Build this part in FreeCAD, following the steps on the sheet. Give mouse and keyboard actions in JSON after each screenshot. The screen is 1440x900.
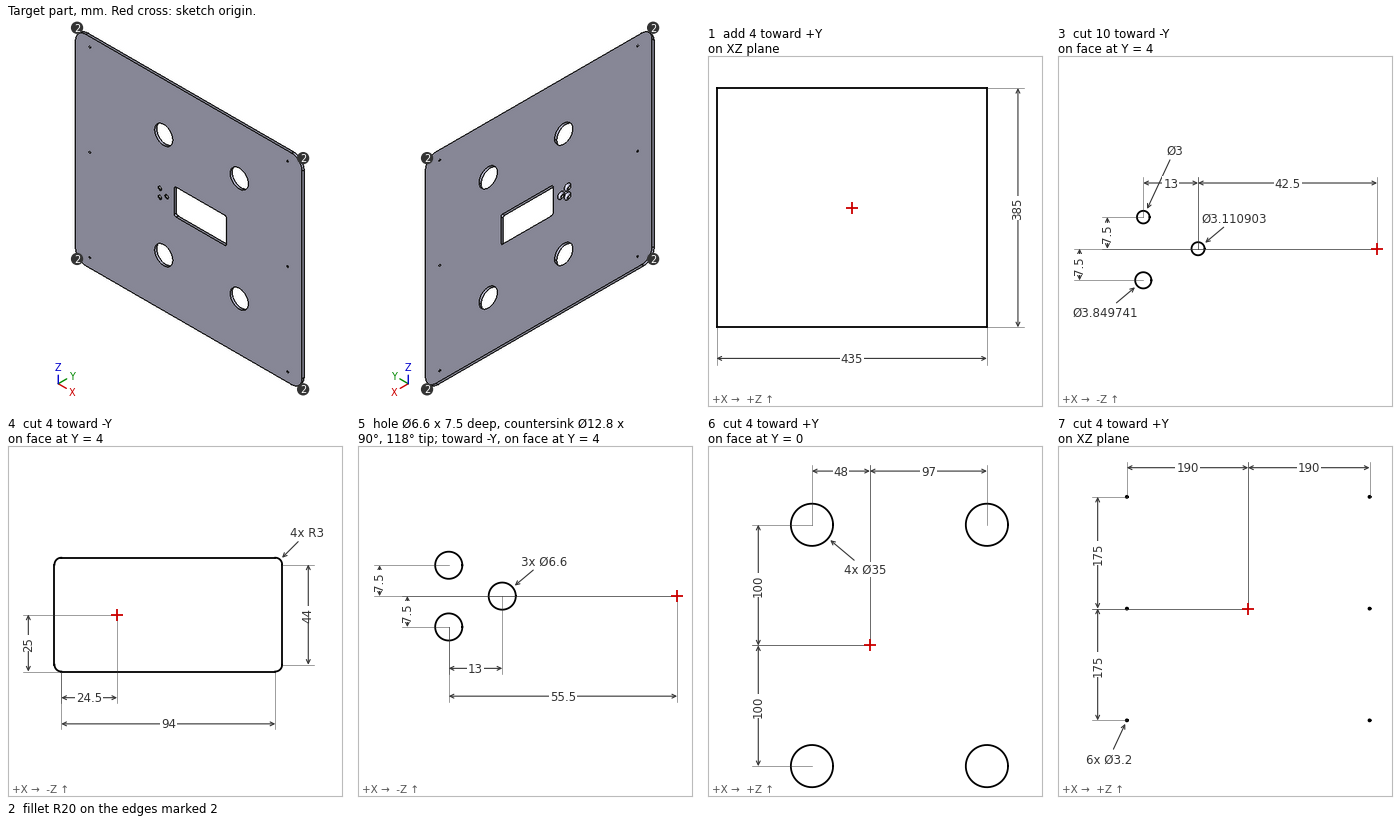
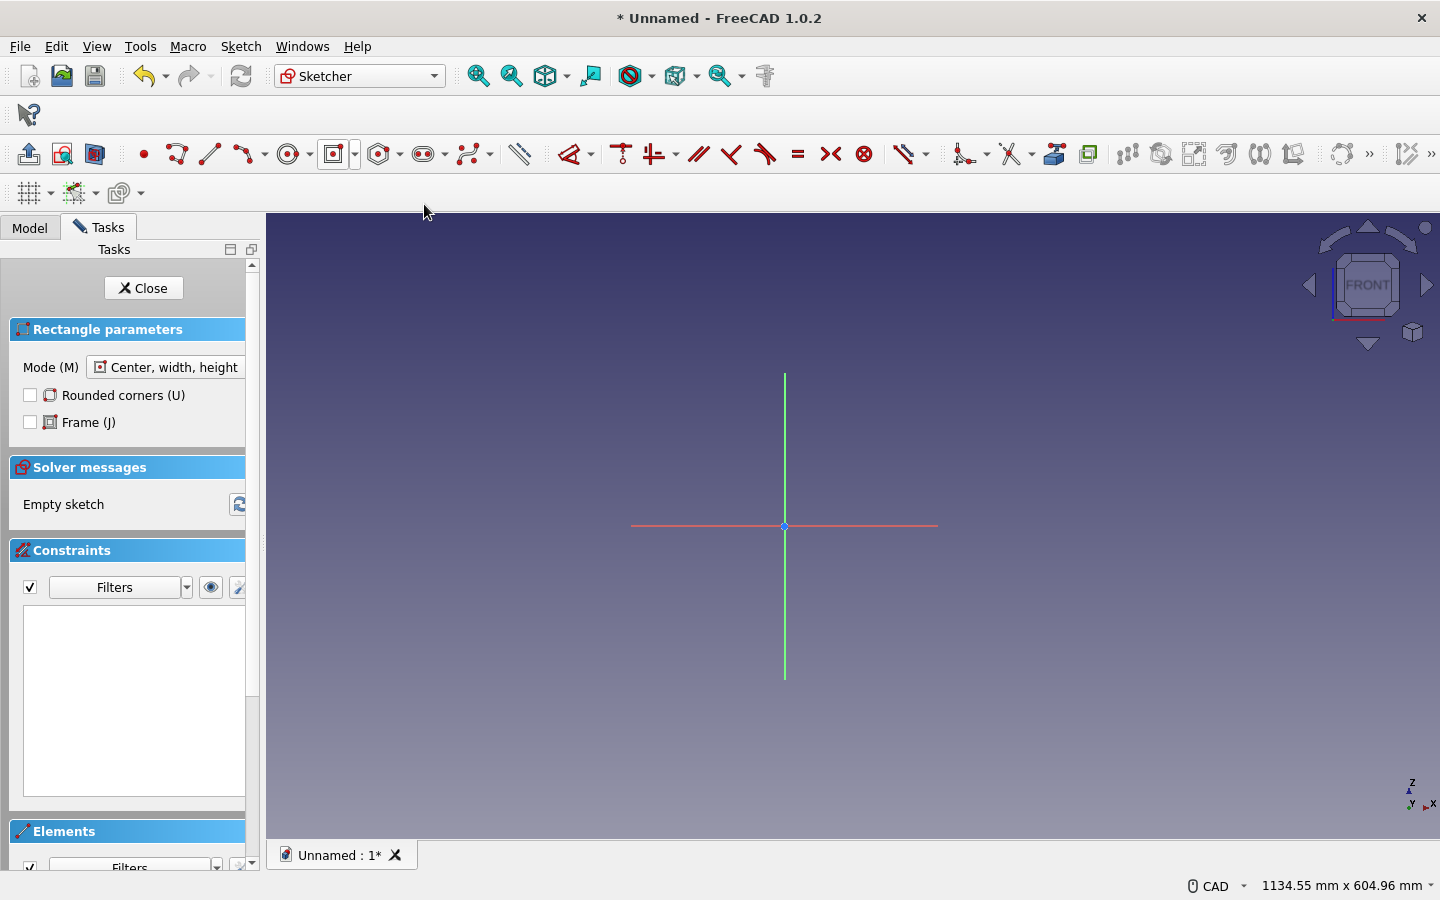
{"action": "left_click", "coordinate": [785, 526]}
{"action": "left_click", "coordinate": [1010, 327]}
{"action": "key", "text": "Escape"}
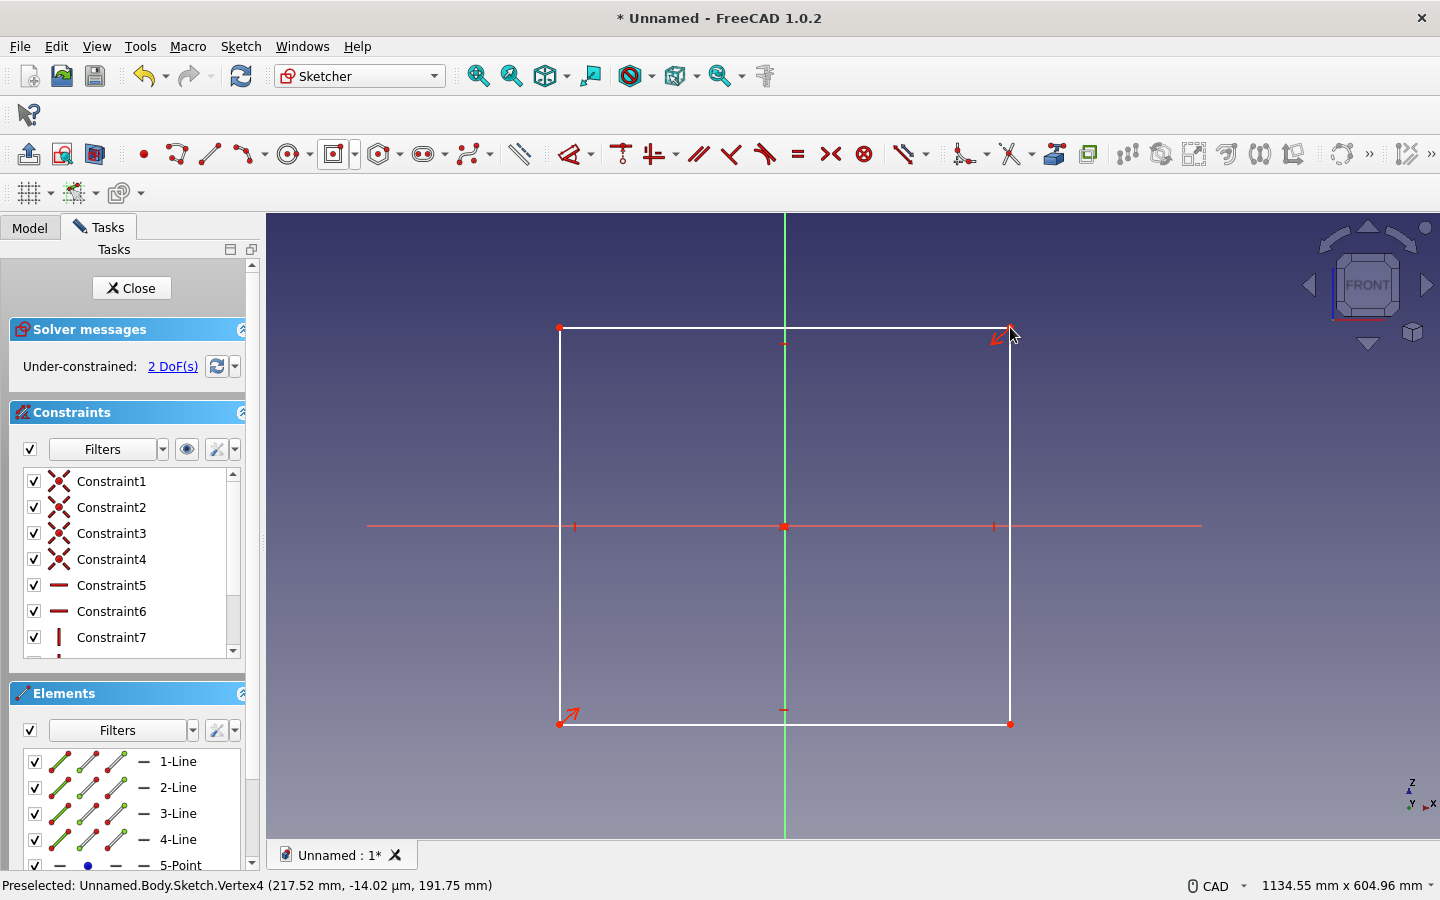
{"action": "left_click", "coordinate": [568, 154]}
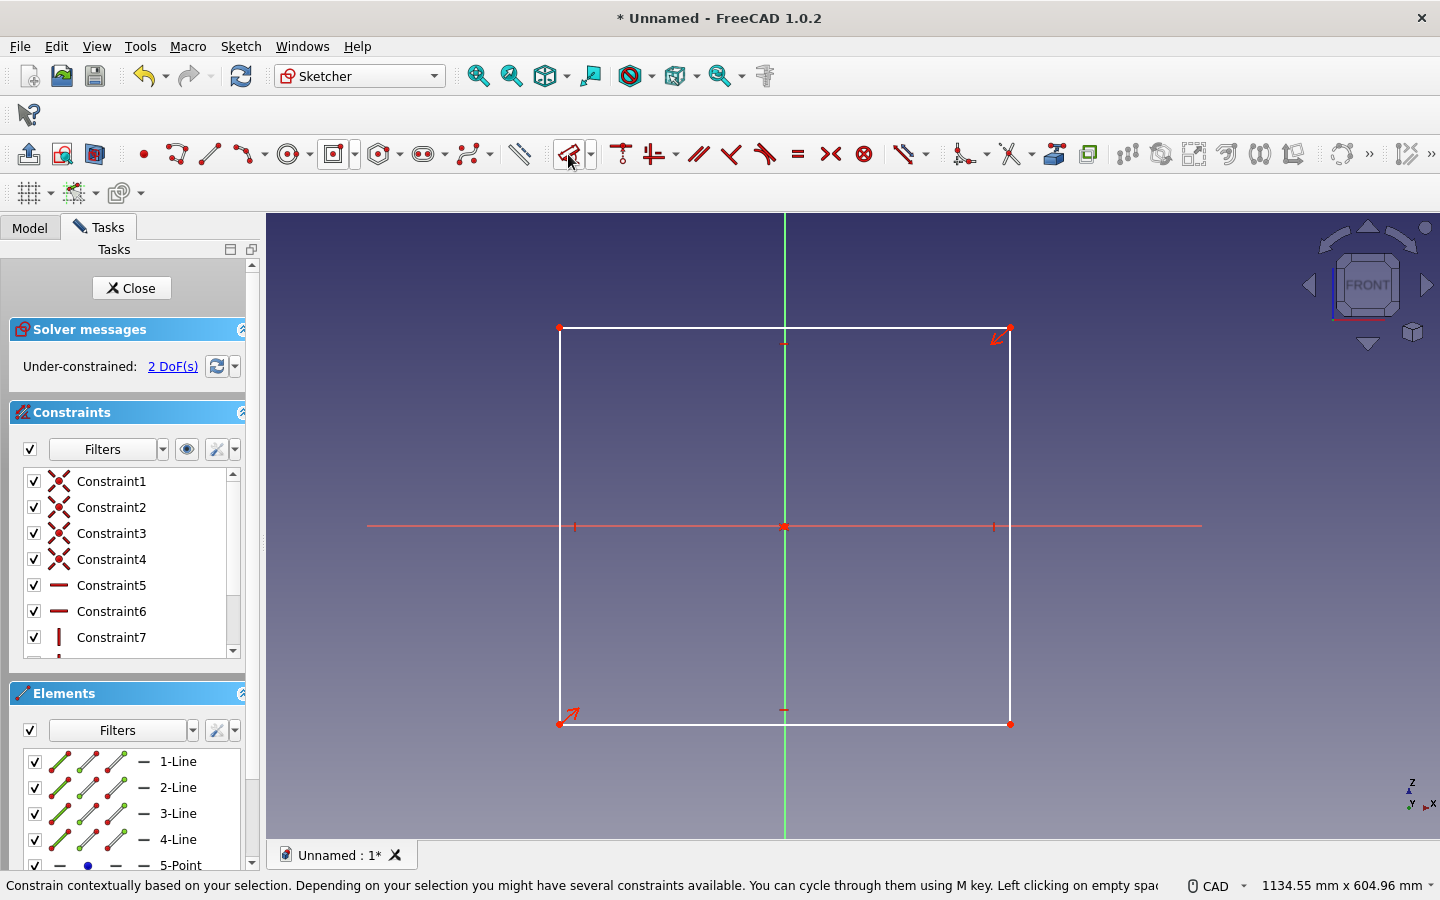
{"action": "left_click", "coordinate": [695, 725]}
{"action": "left_click", "coordinate": [681, 759]}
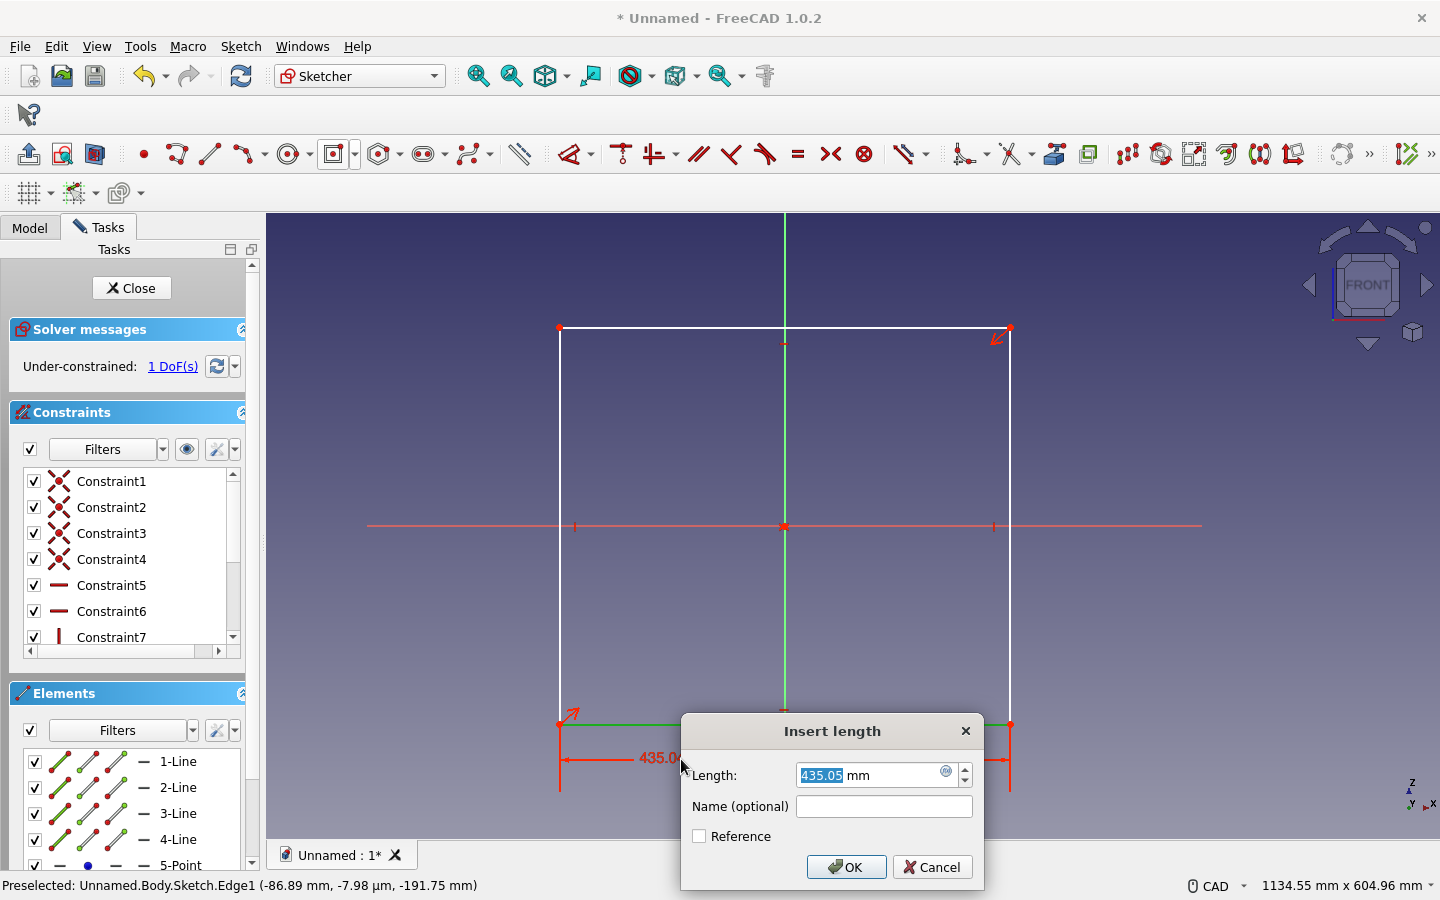
{"action": "type", "text": "435"}
{"action": "key", "text": "Return"}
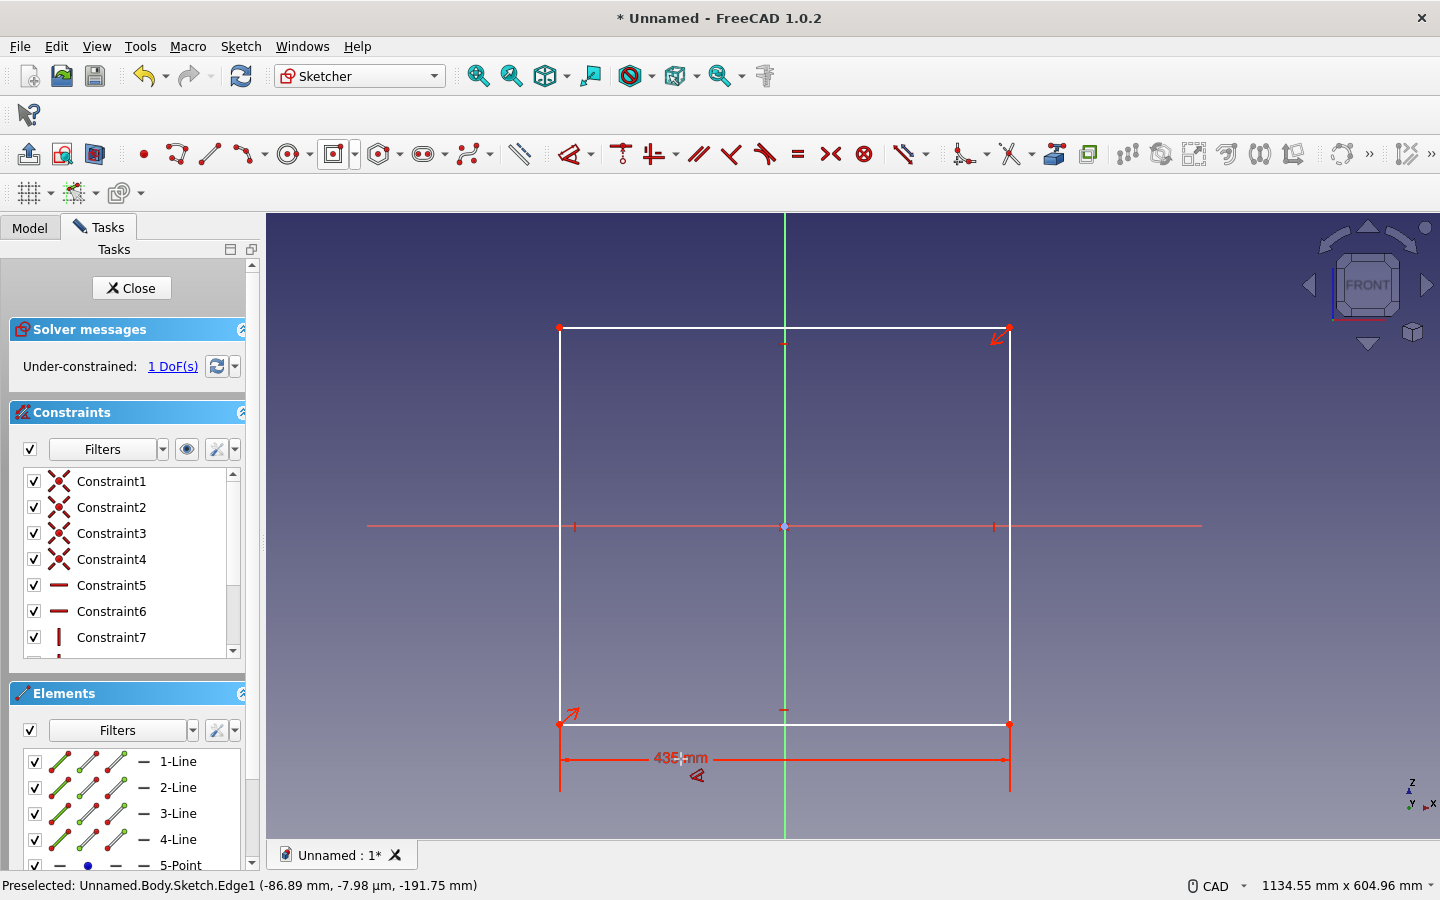
{"action": "left_click", "coordinate": [1010, 606]}
{"action": "left_click", "coordinate": [1044, 435]}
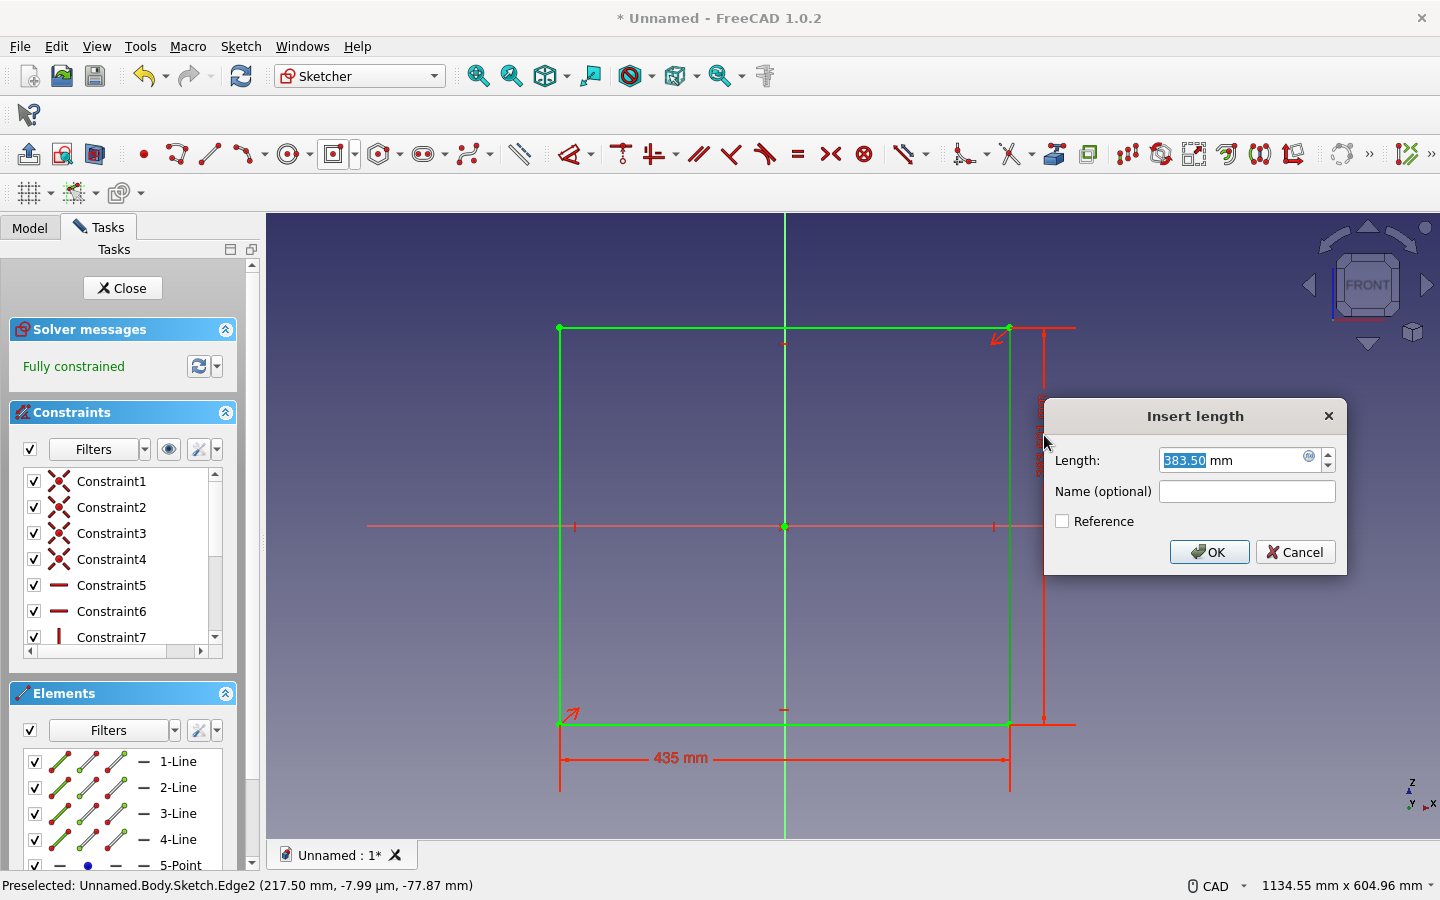
{"action": "type", "text": "385"}
{"action": "key", "text": "Return"}
{"action": "key", "text": "Escape"}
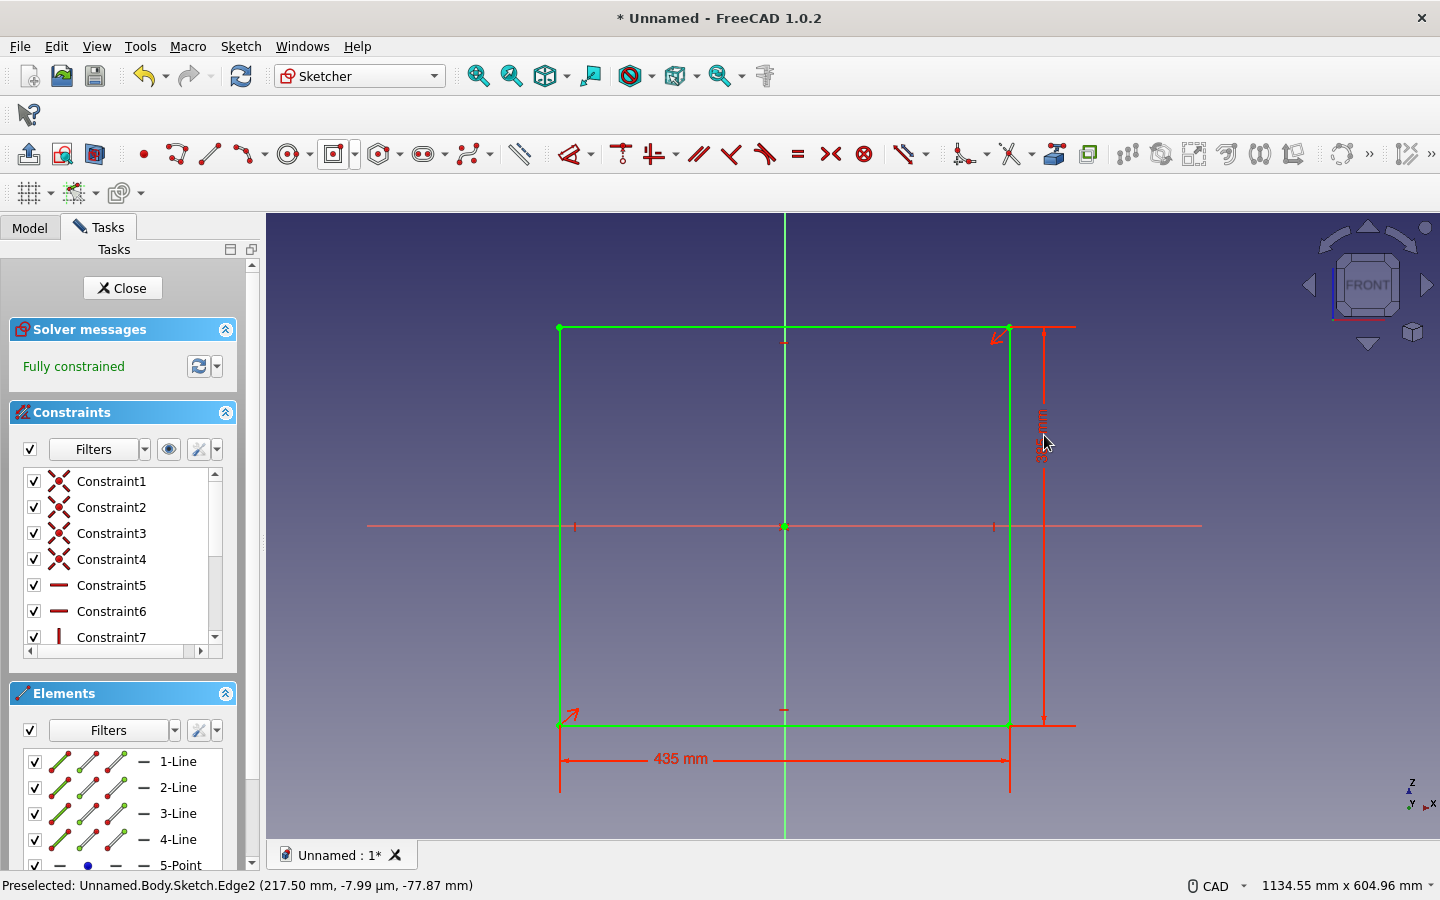
{"action": "left_click", "coordinate": [123, 288]}